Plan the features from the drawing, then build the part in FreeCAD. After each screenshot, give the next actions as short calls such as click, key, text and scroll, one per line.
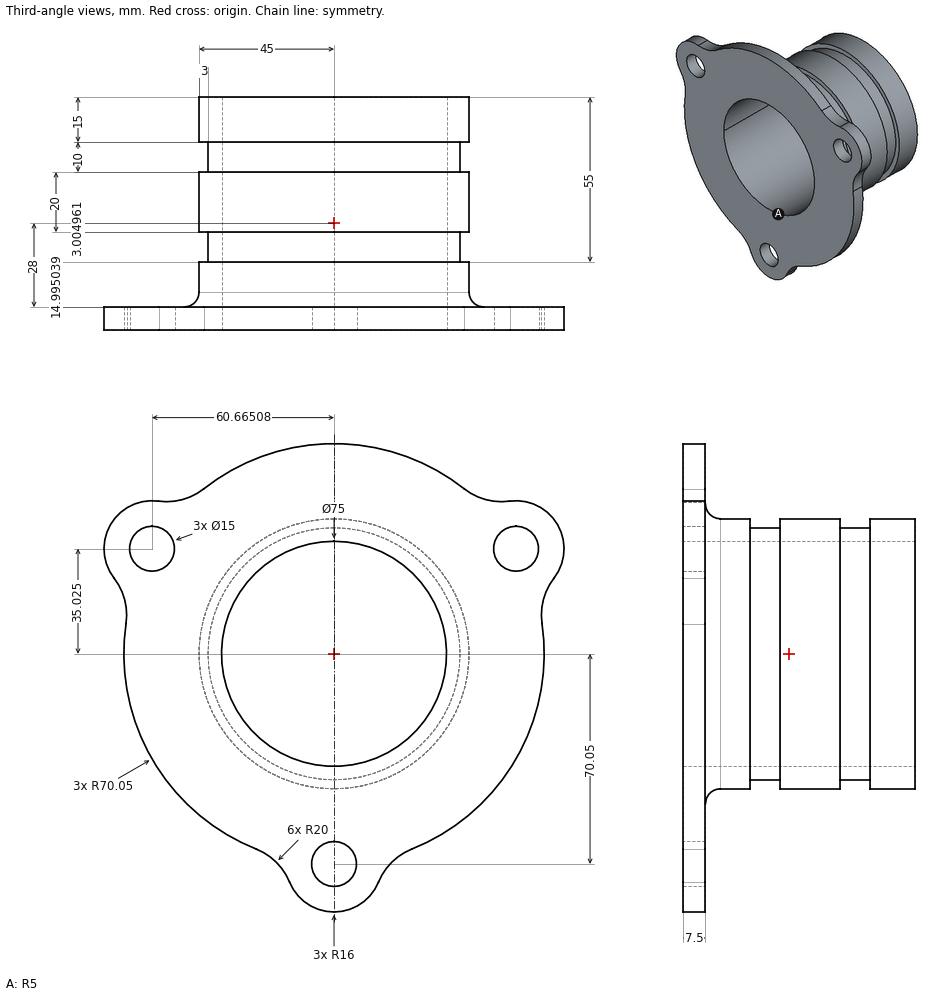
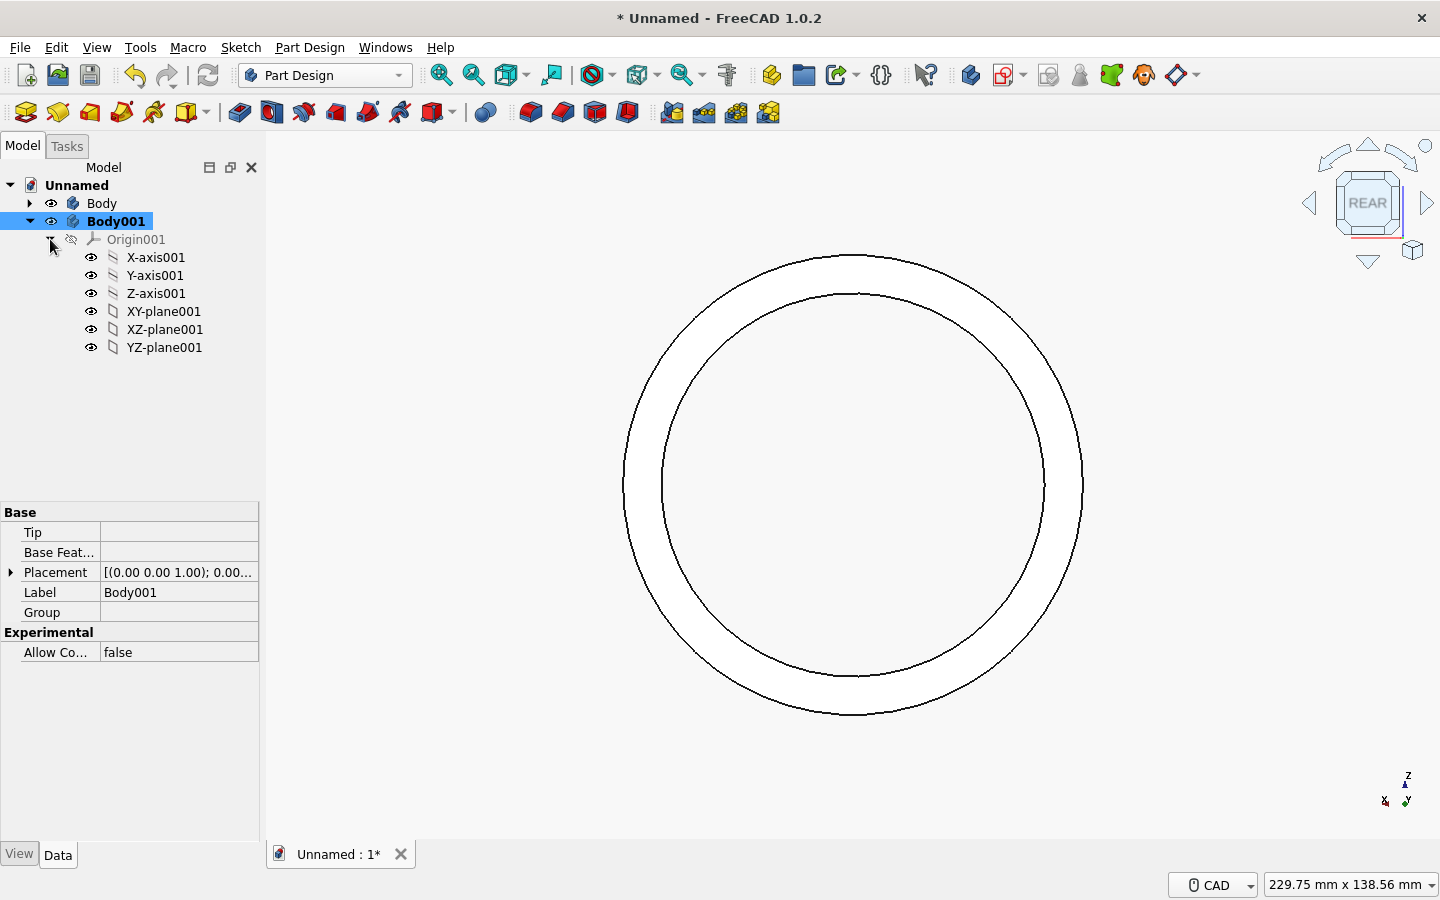
click(136, 329)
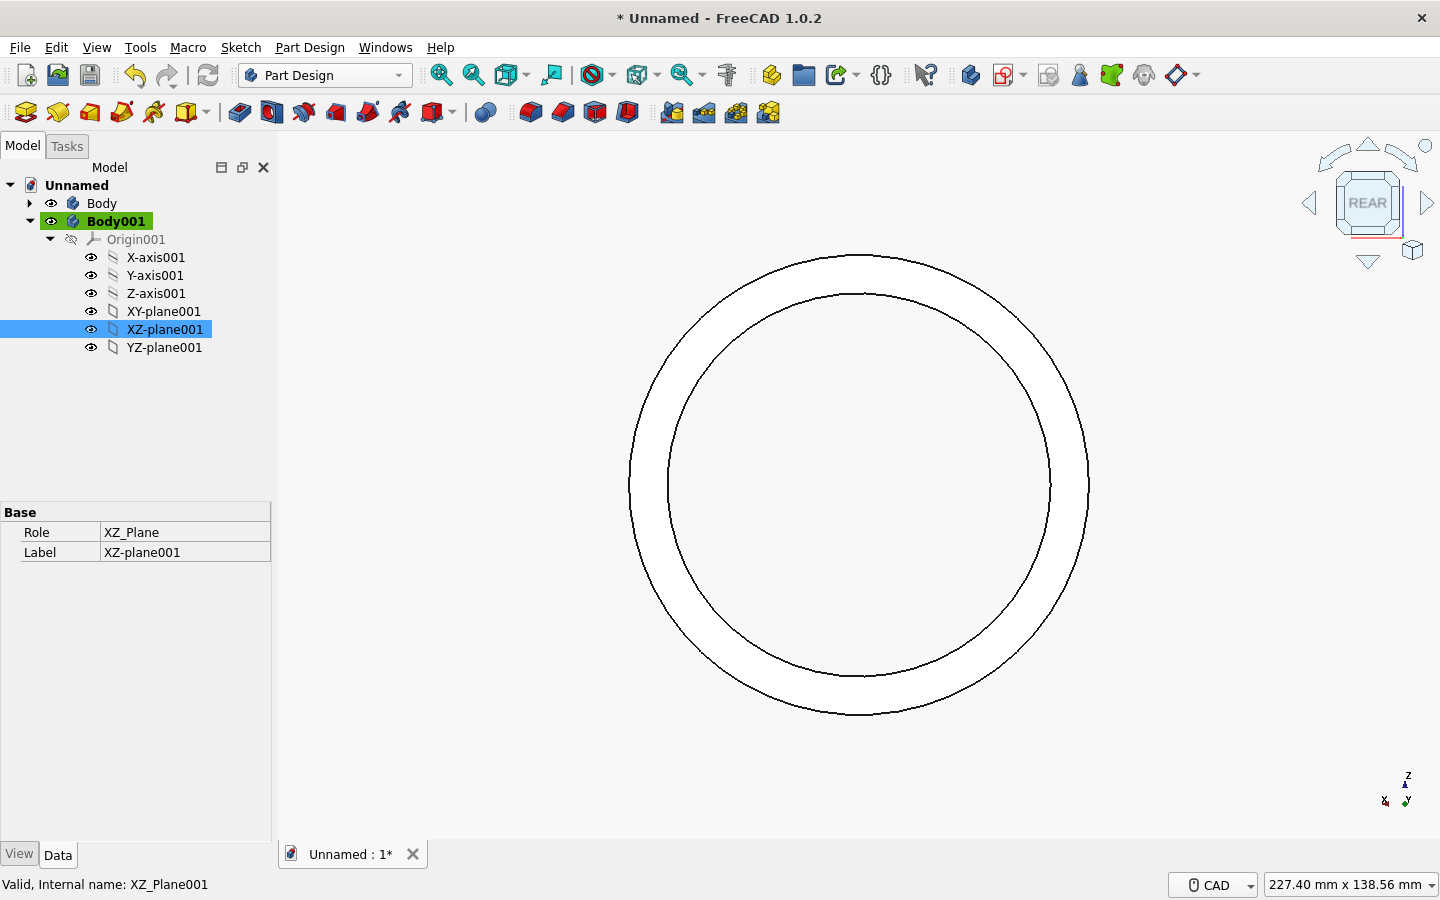
click(1176, 76)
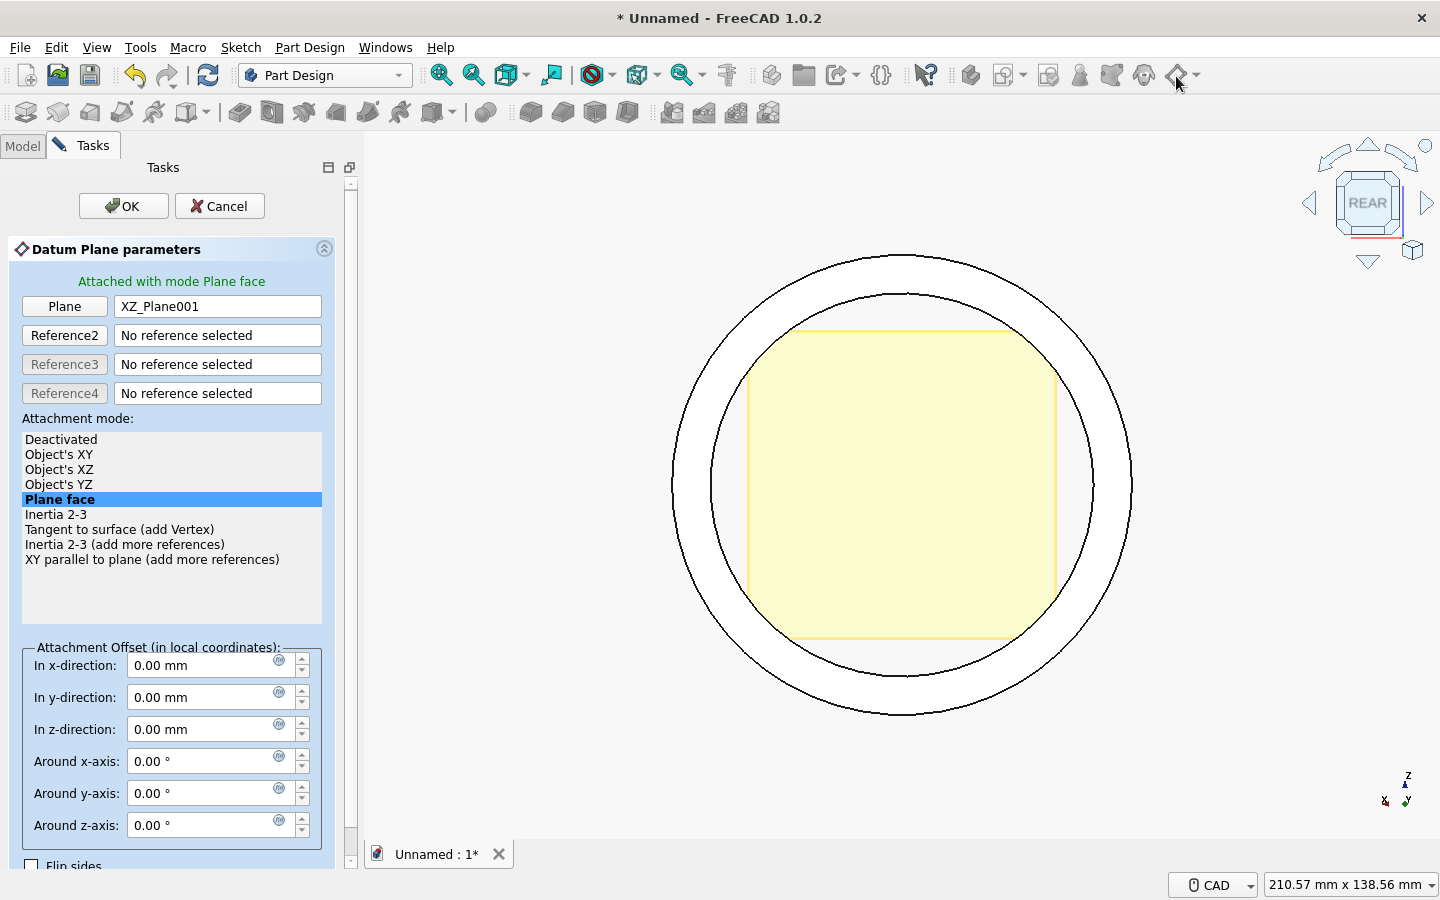
triple_click(210, 729)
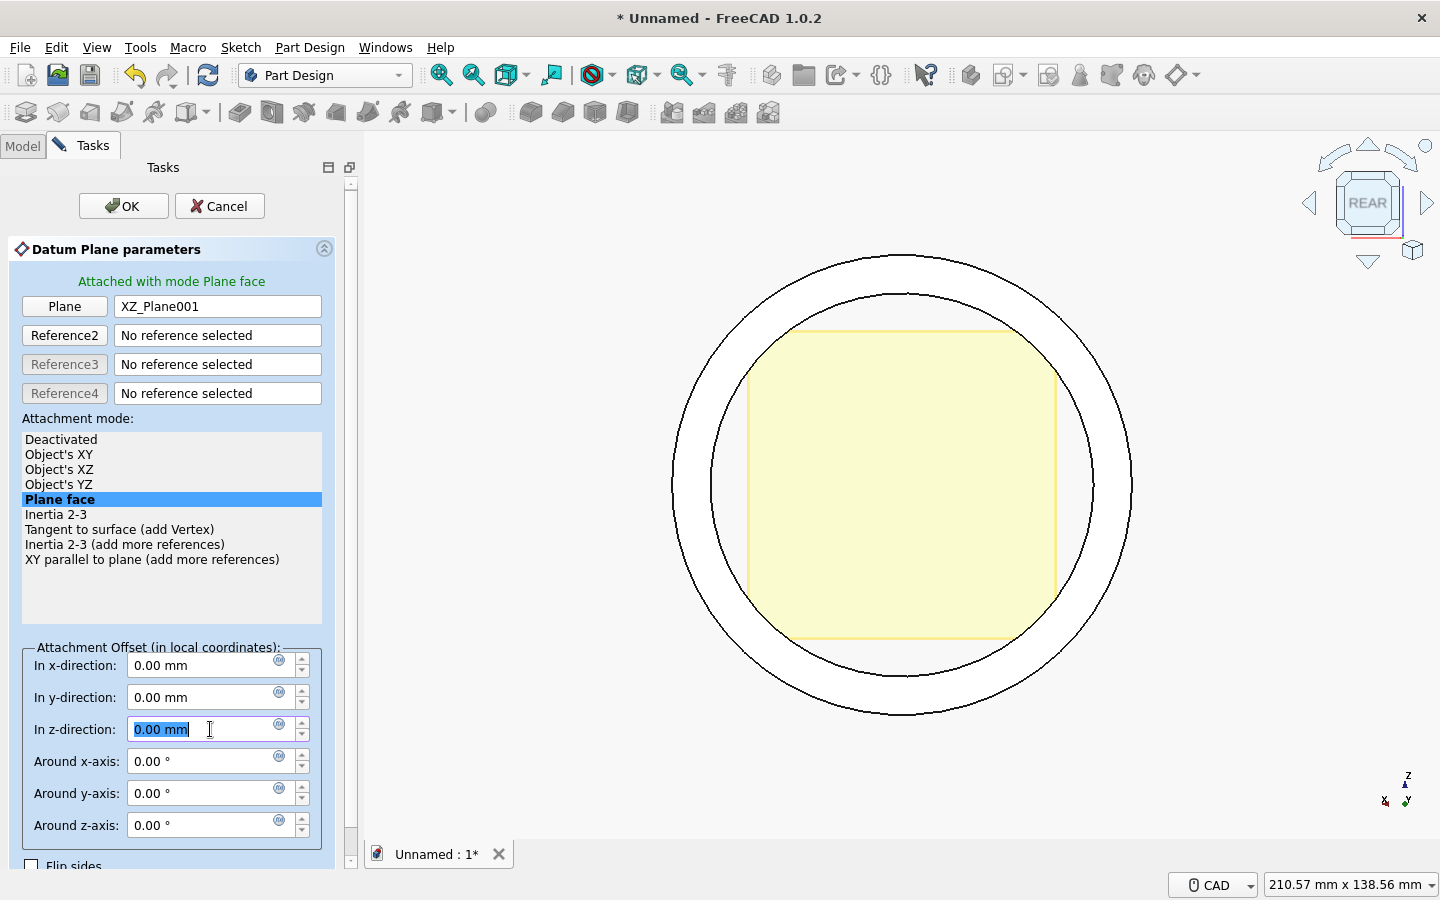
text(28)
key(Tab)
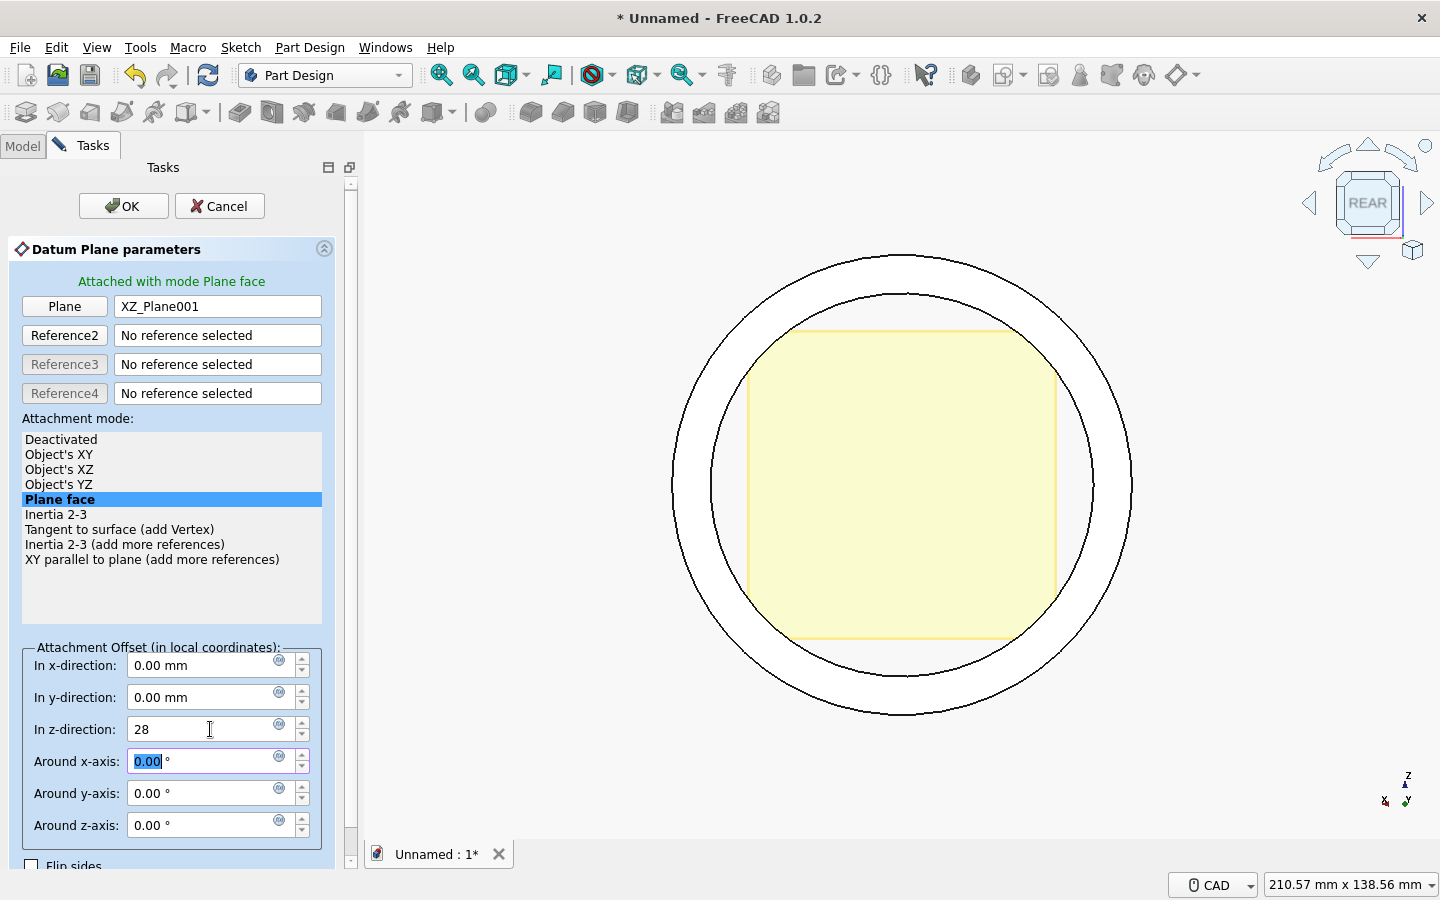
click(124, 206)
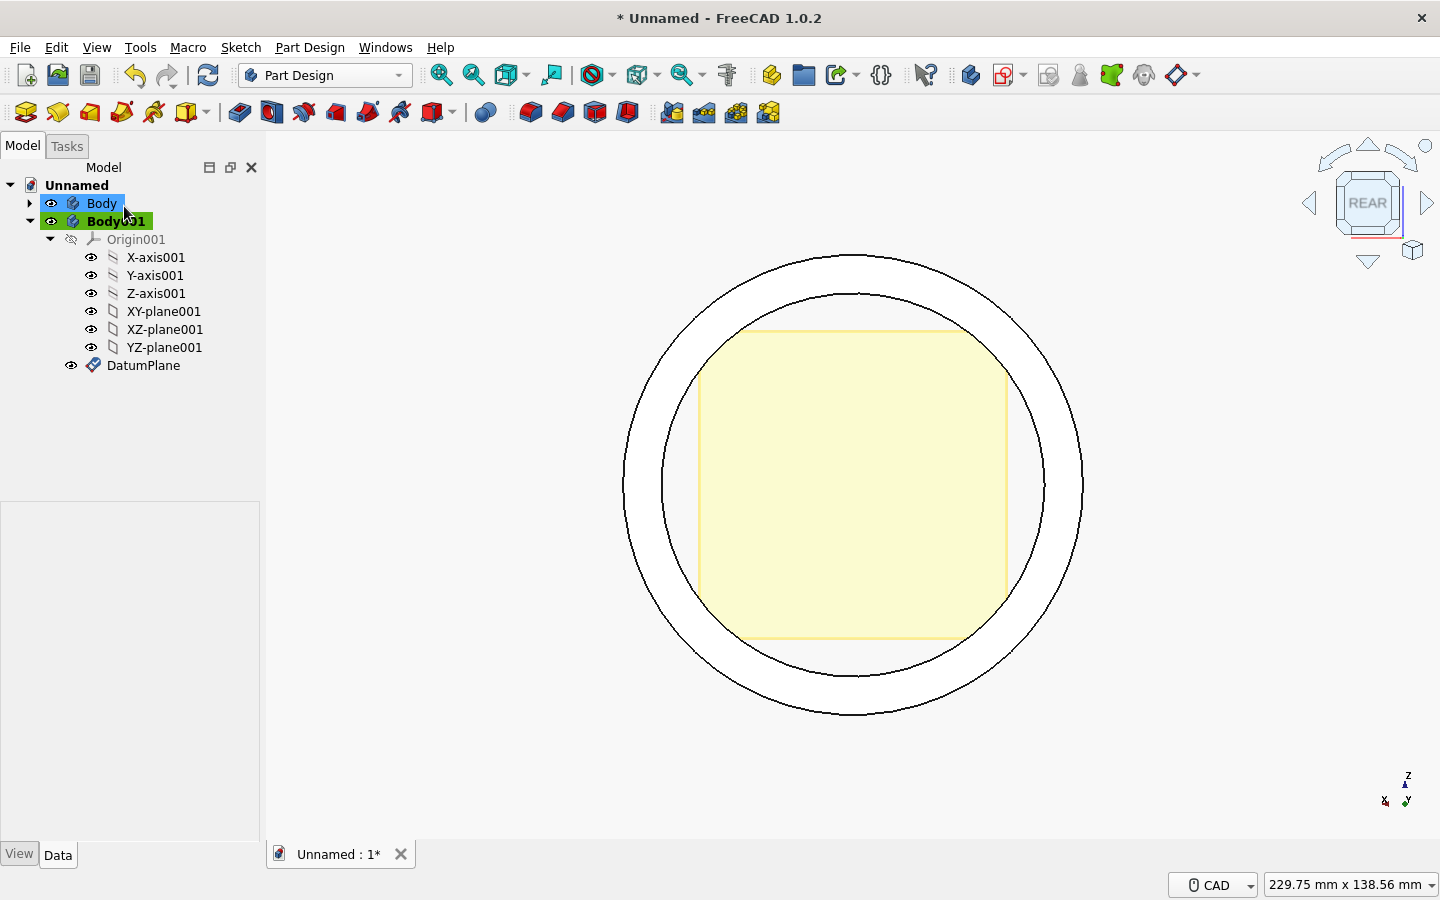
click(116, 365)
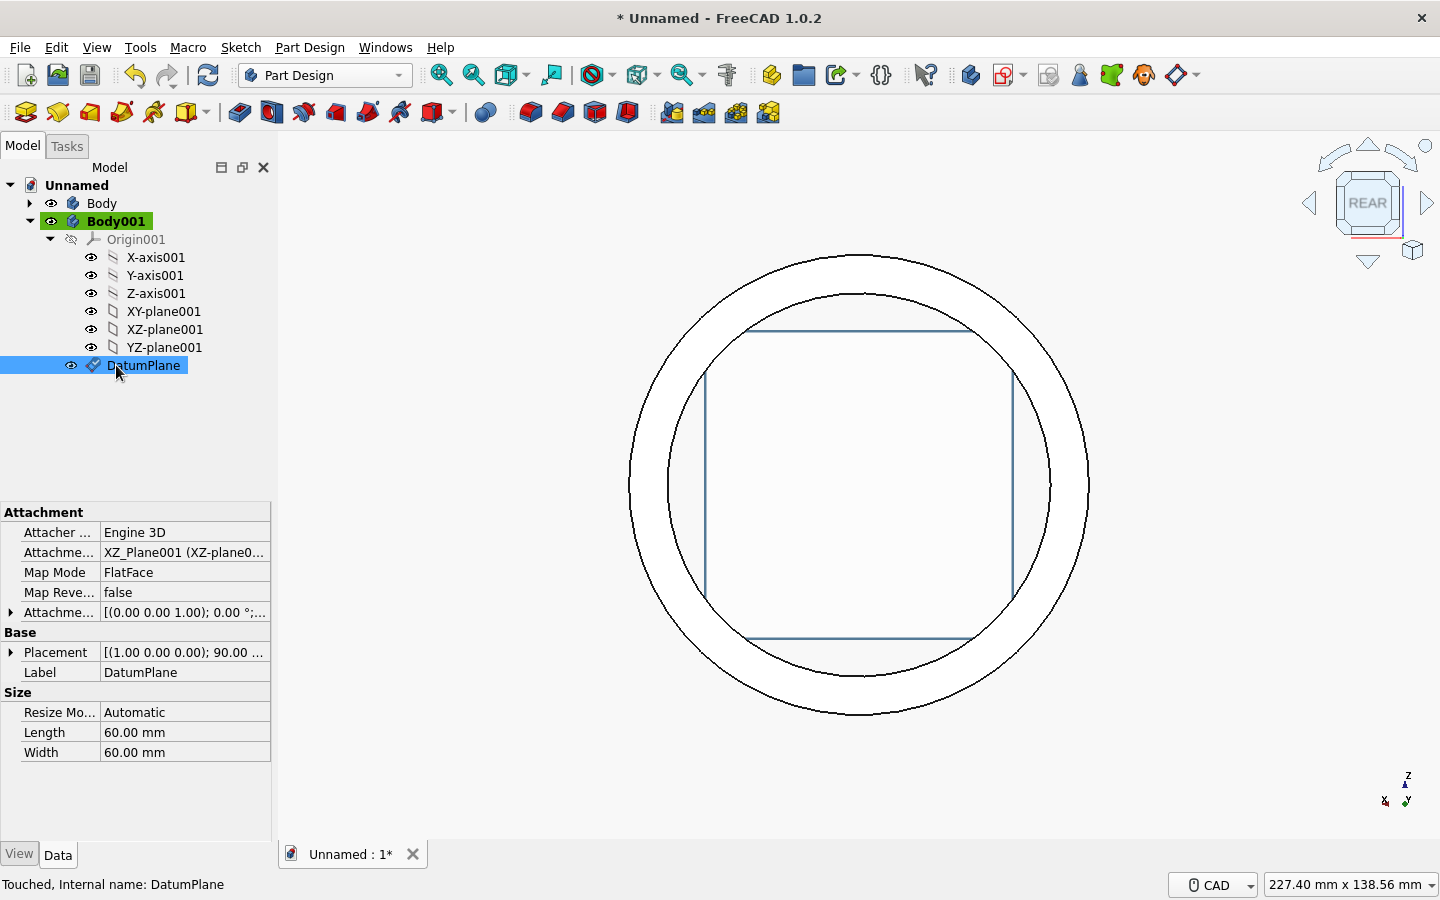
click(1004, 76)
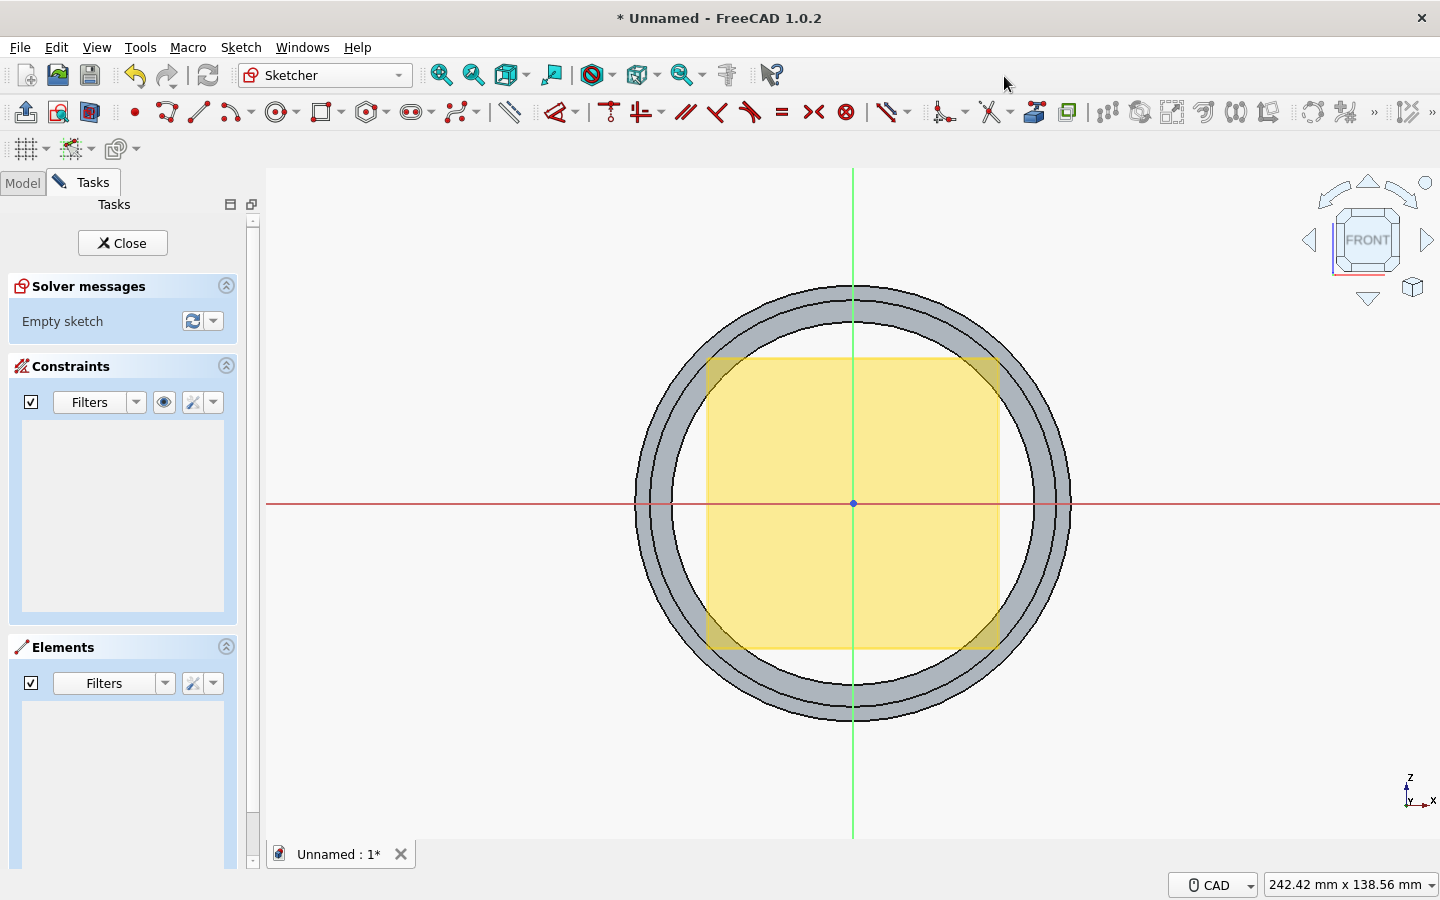
scroll(701, 456, down, 3)